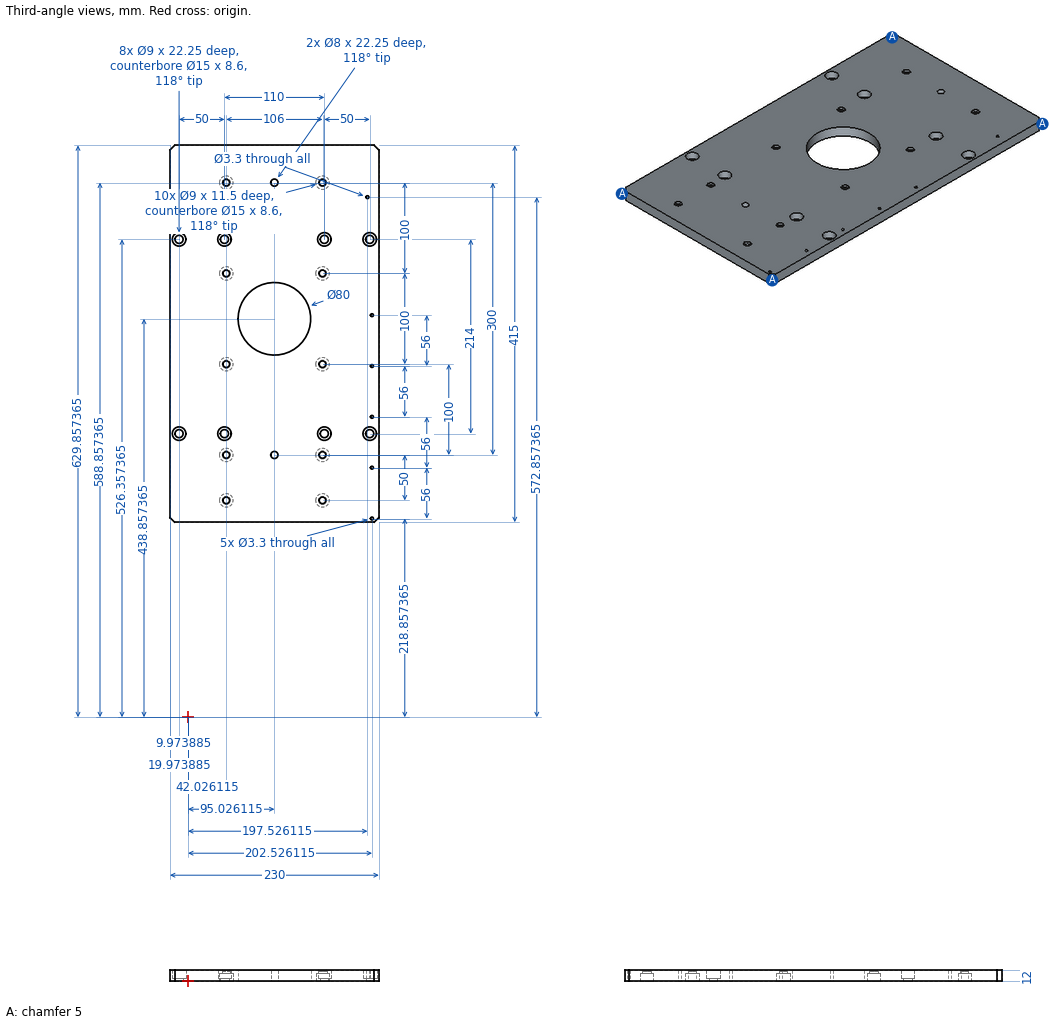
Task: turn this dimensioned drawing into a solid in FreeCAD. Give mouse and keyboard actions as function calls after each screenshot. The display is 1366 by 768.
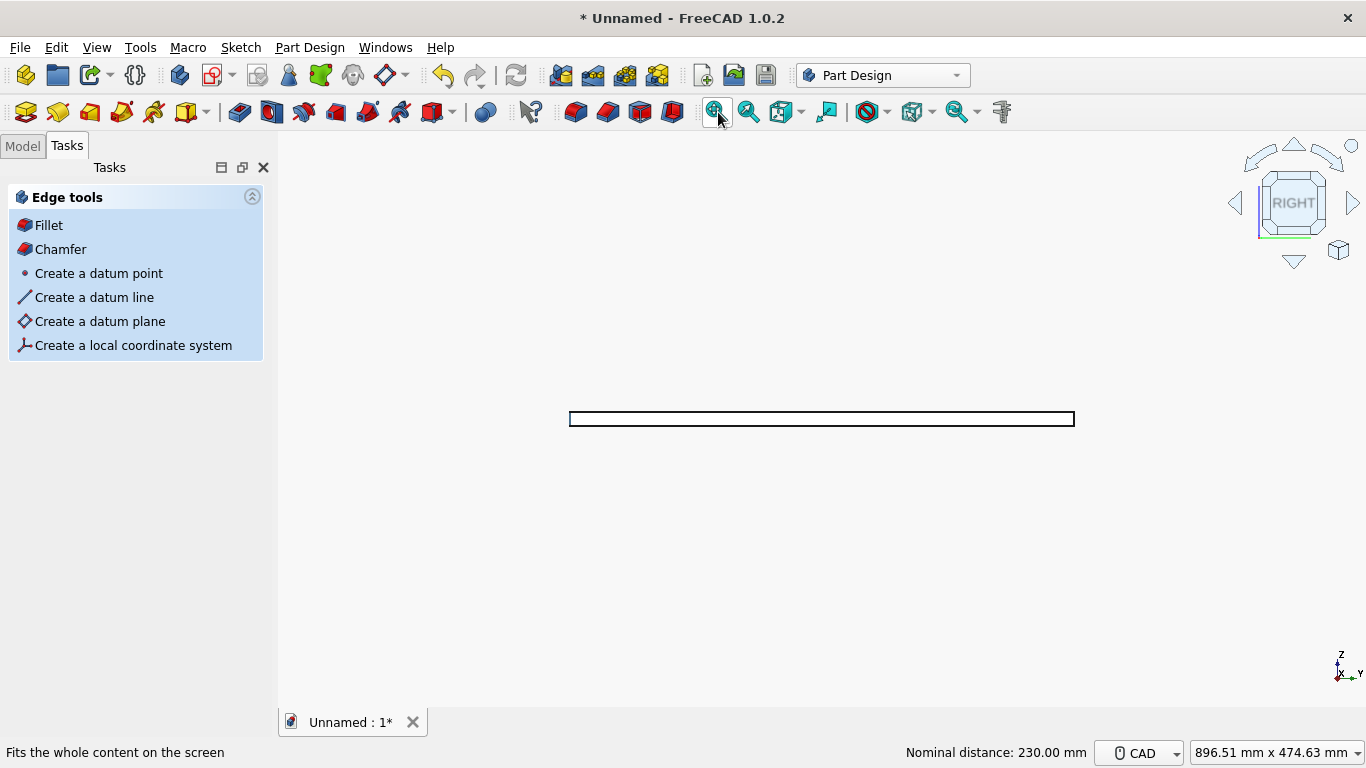
click(1074, 418, ctrl)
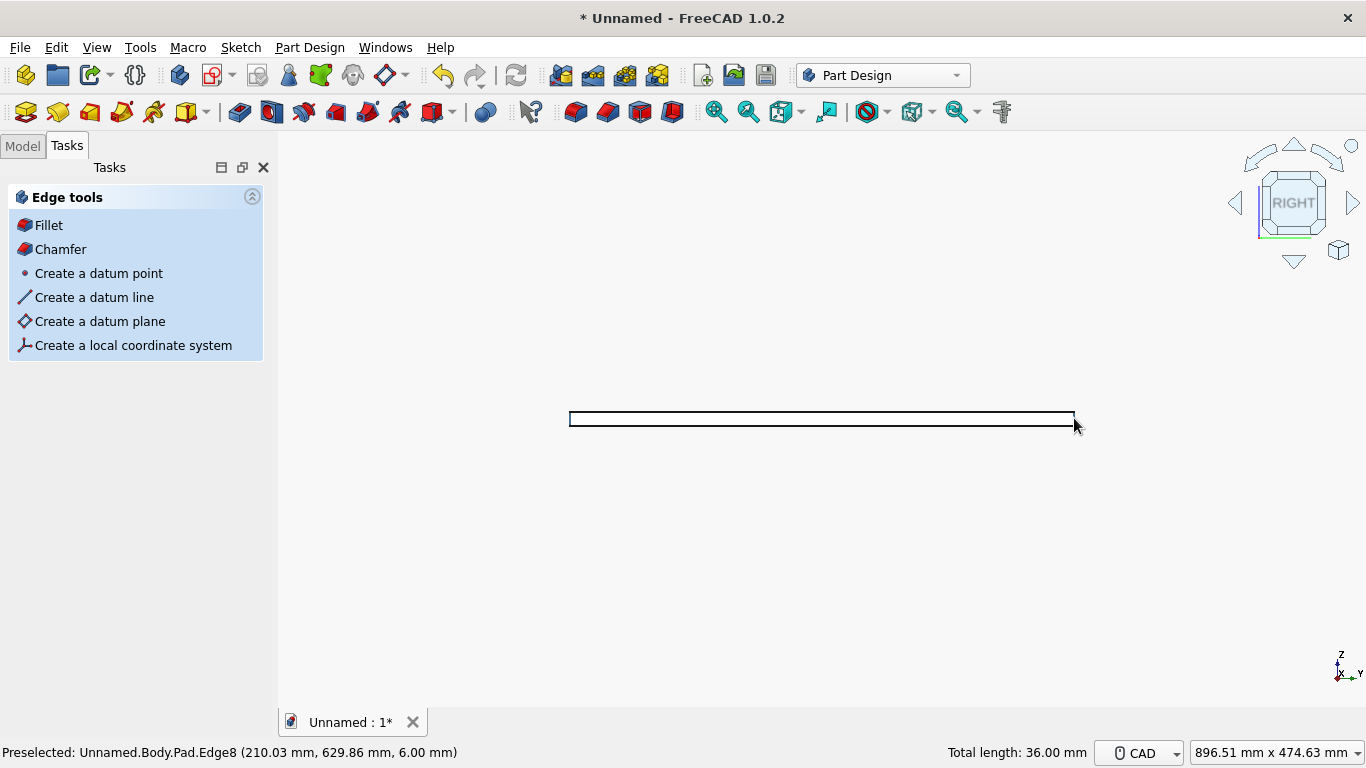
scroll(1074, 418, up, 6)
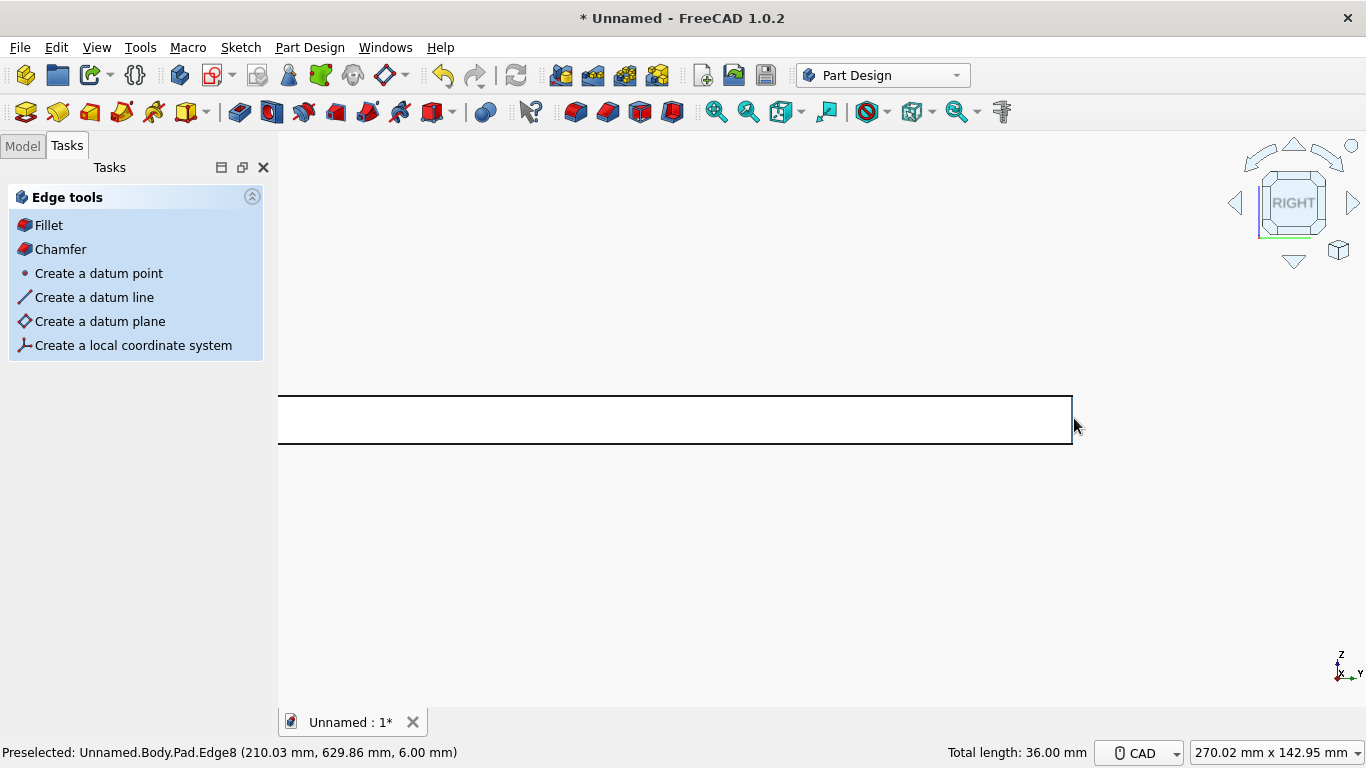
click(718, 112)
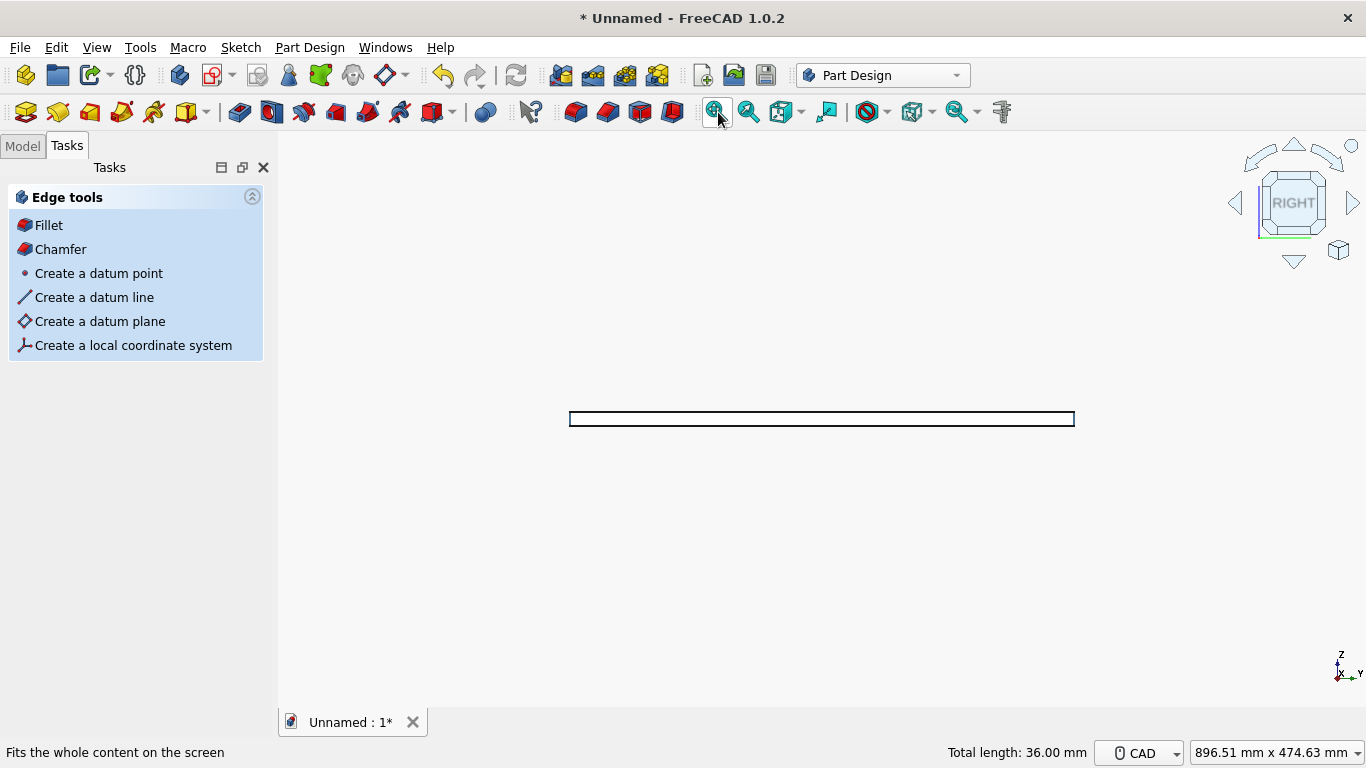
key(5)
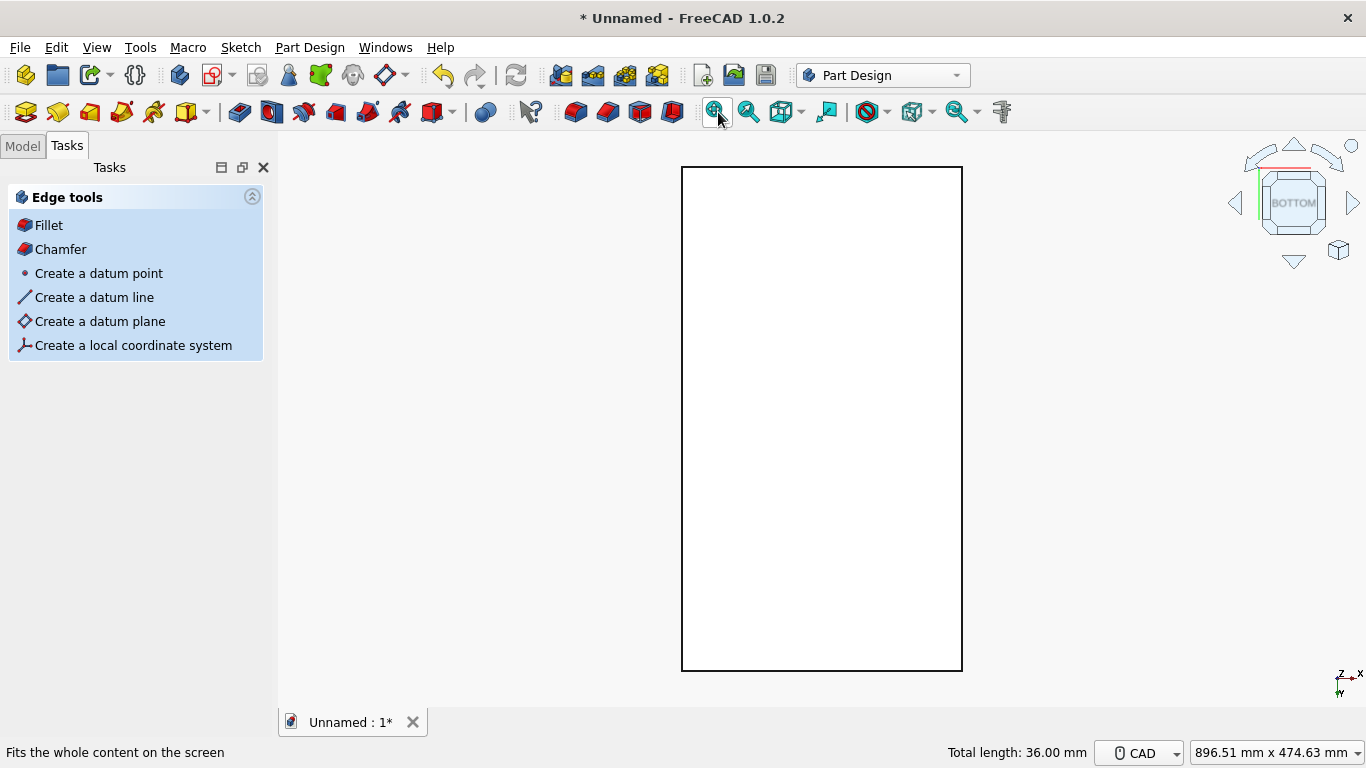
scroll(682, 670, up, 6)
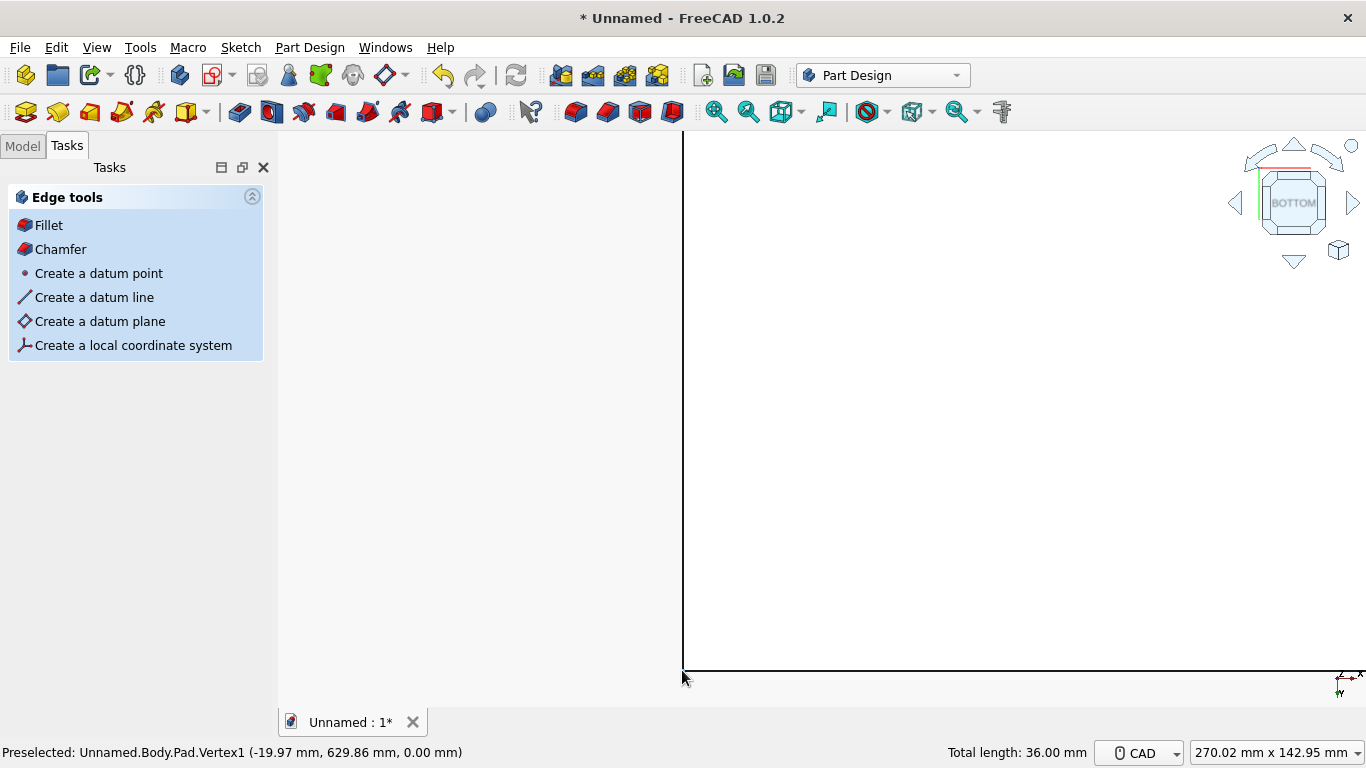
click(718, 112)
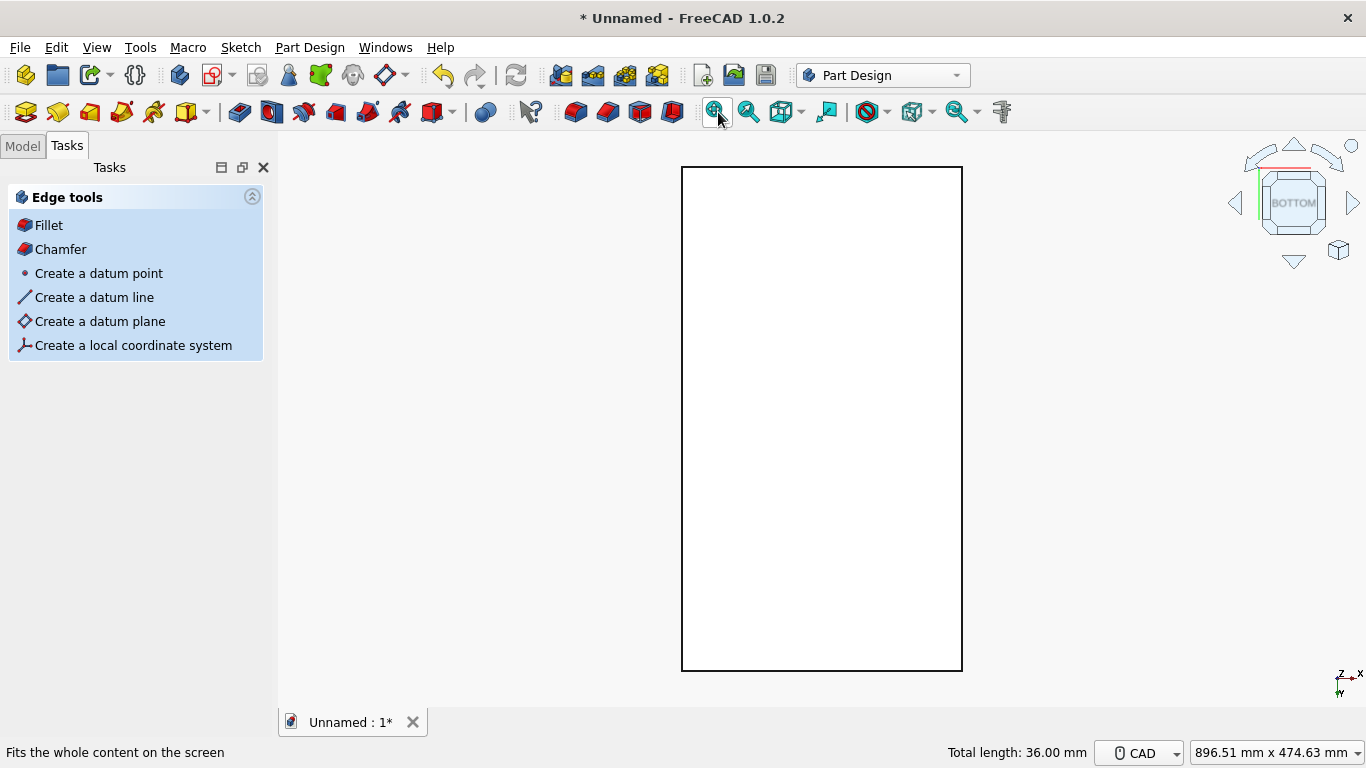
key(4)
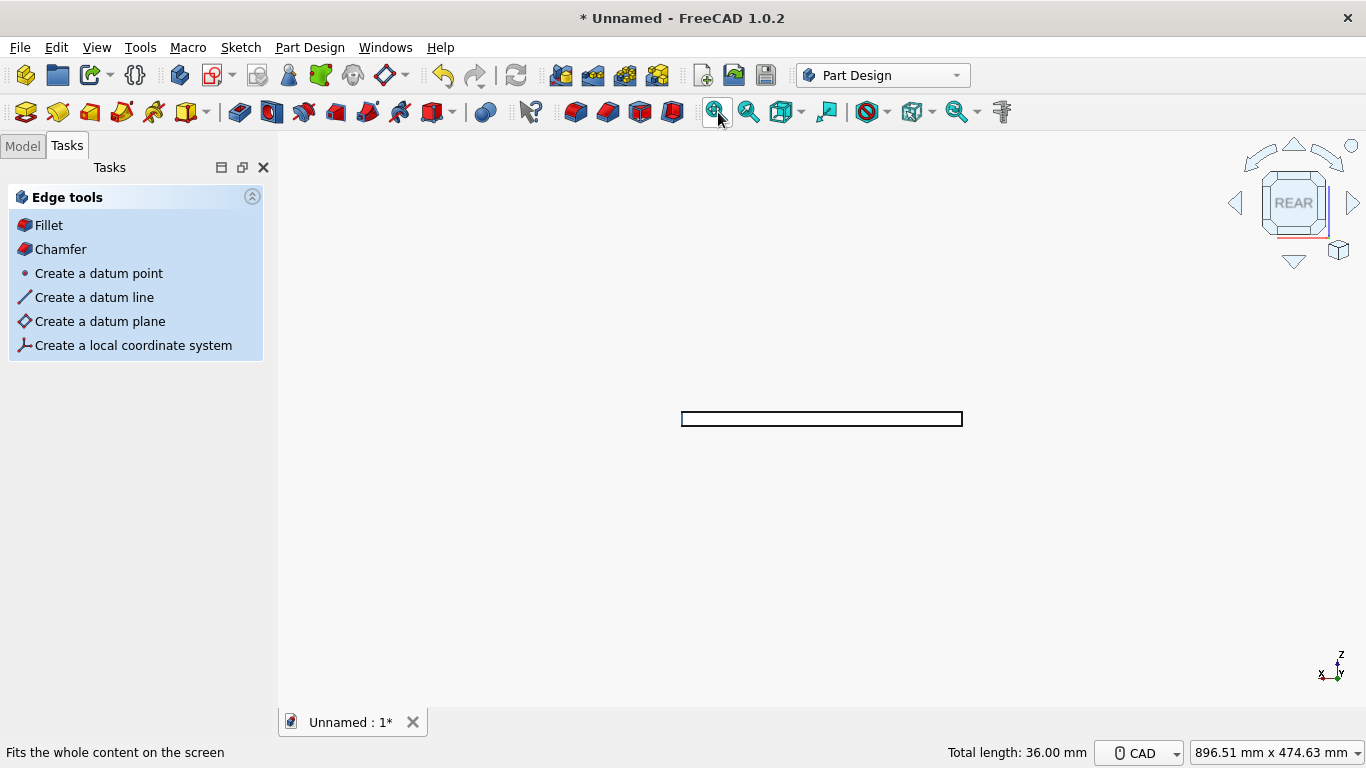
click(718, 112)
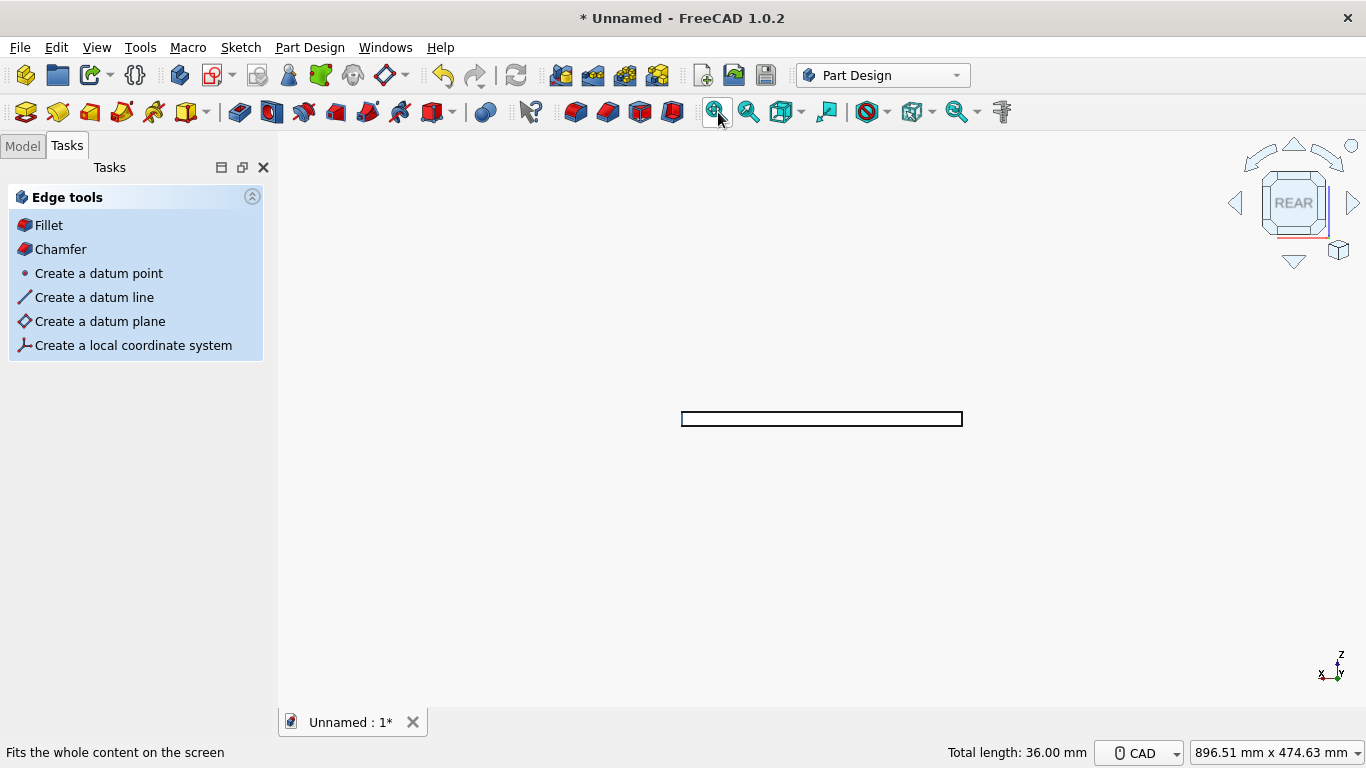
click(962, 418, ctrl)